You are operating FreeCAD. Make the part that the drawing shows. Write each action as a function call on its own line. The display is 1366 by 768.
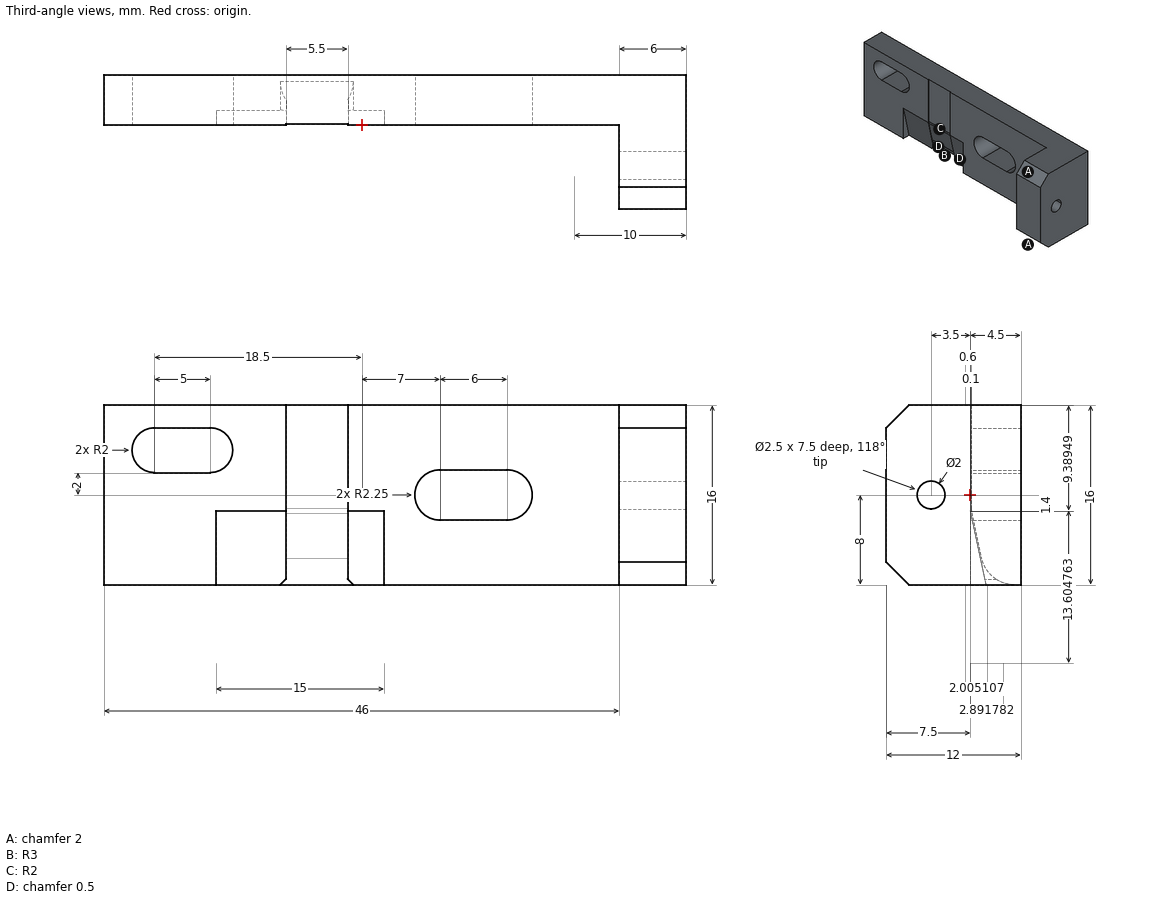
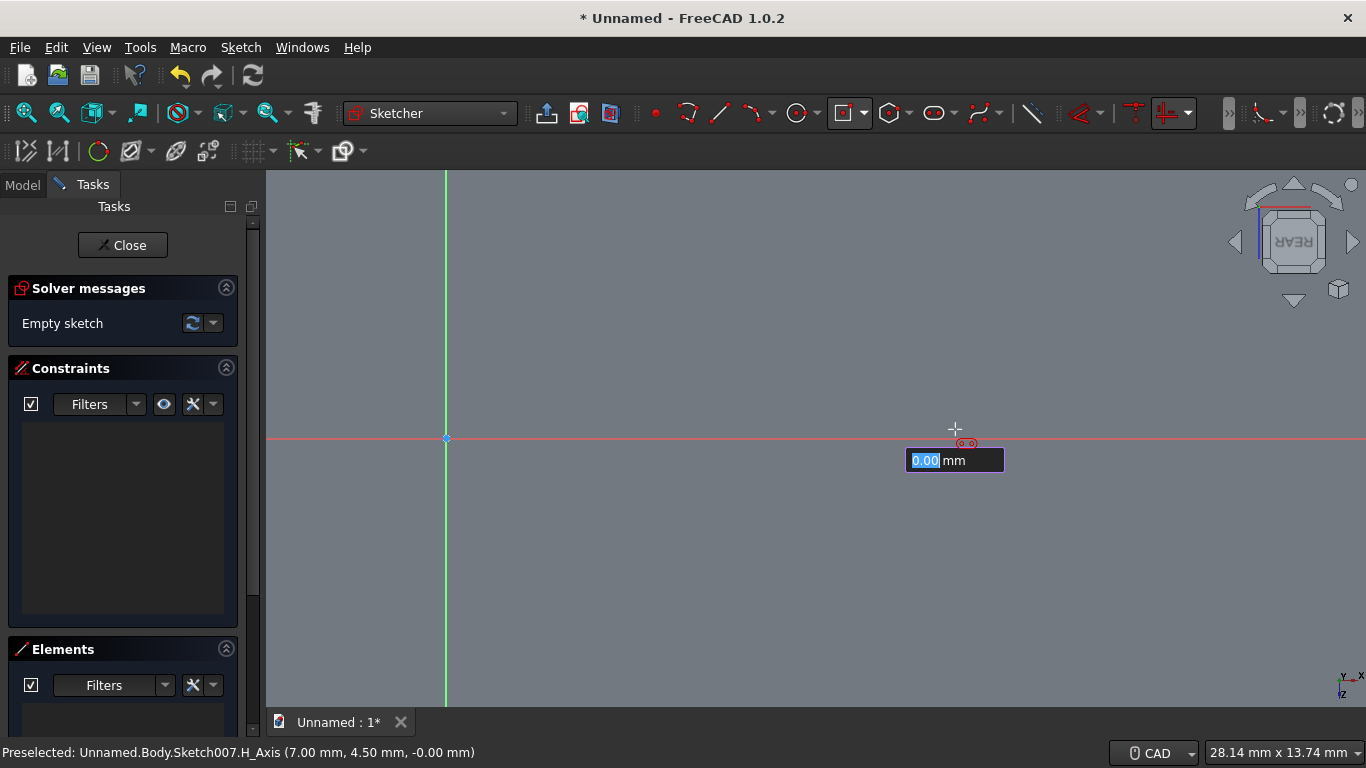
click(837, 351)
key(Escape)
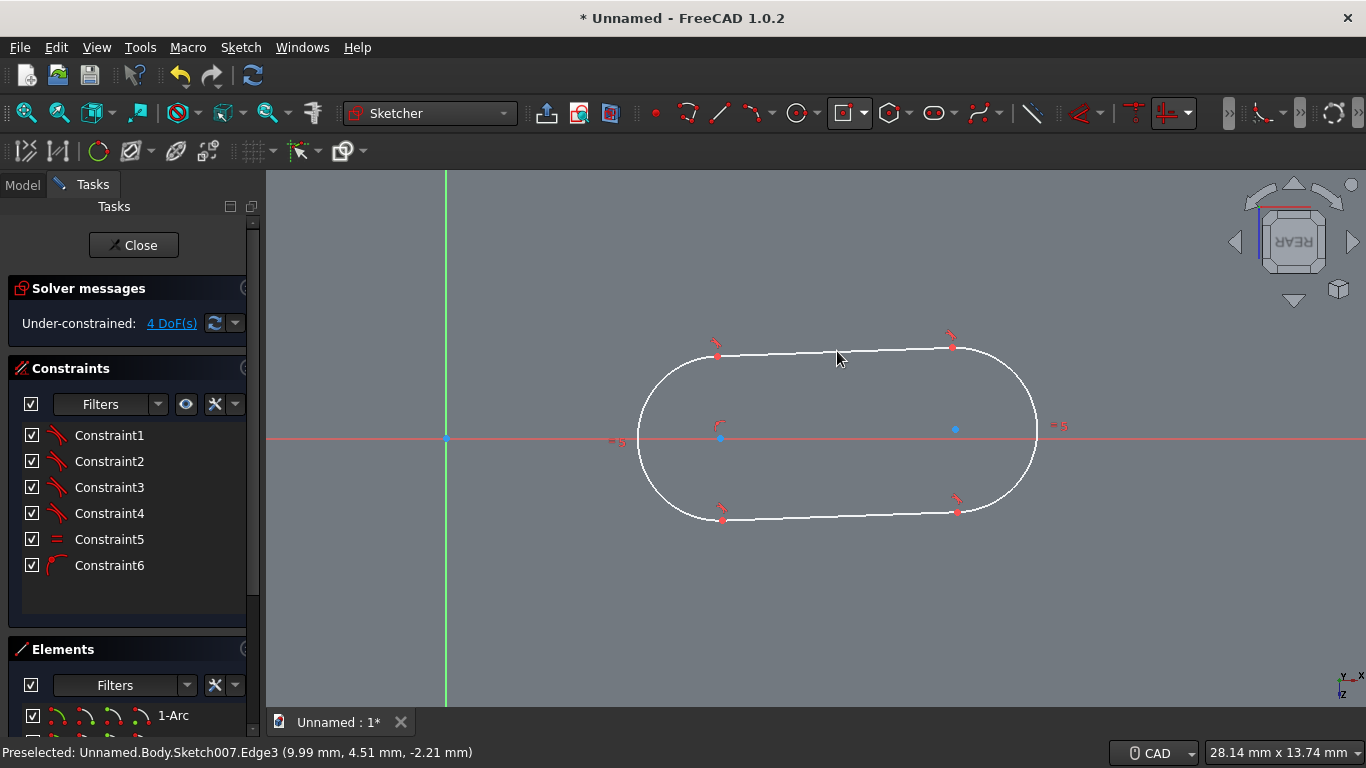
click(788, 354)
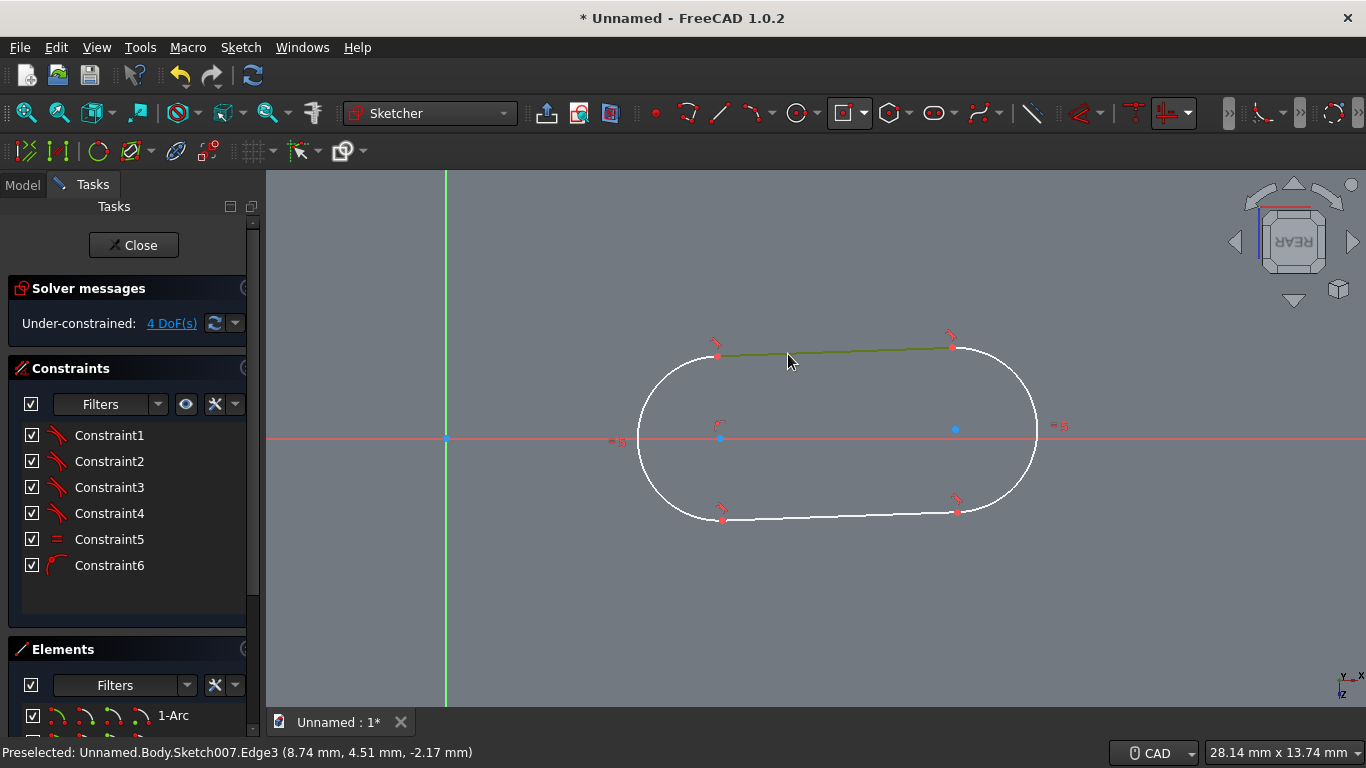
key(h)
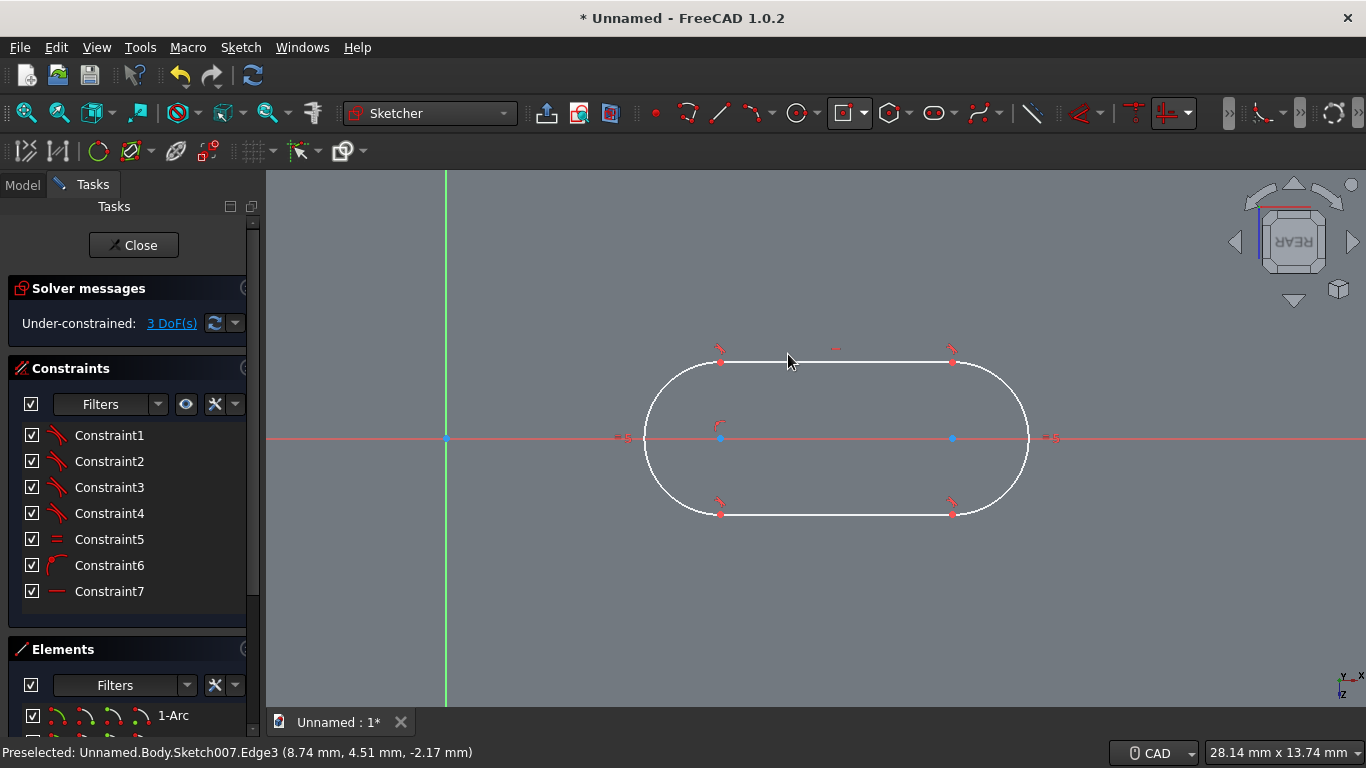
key(d)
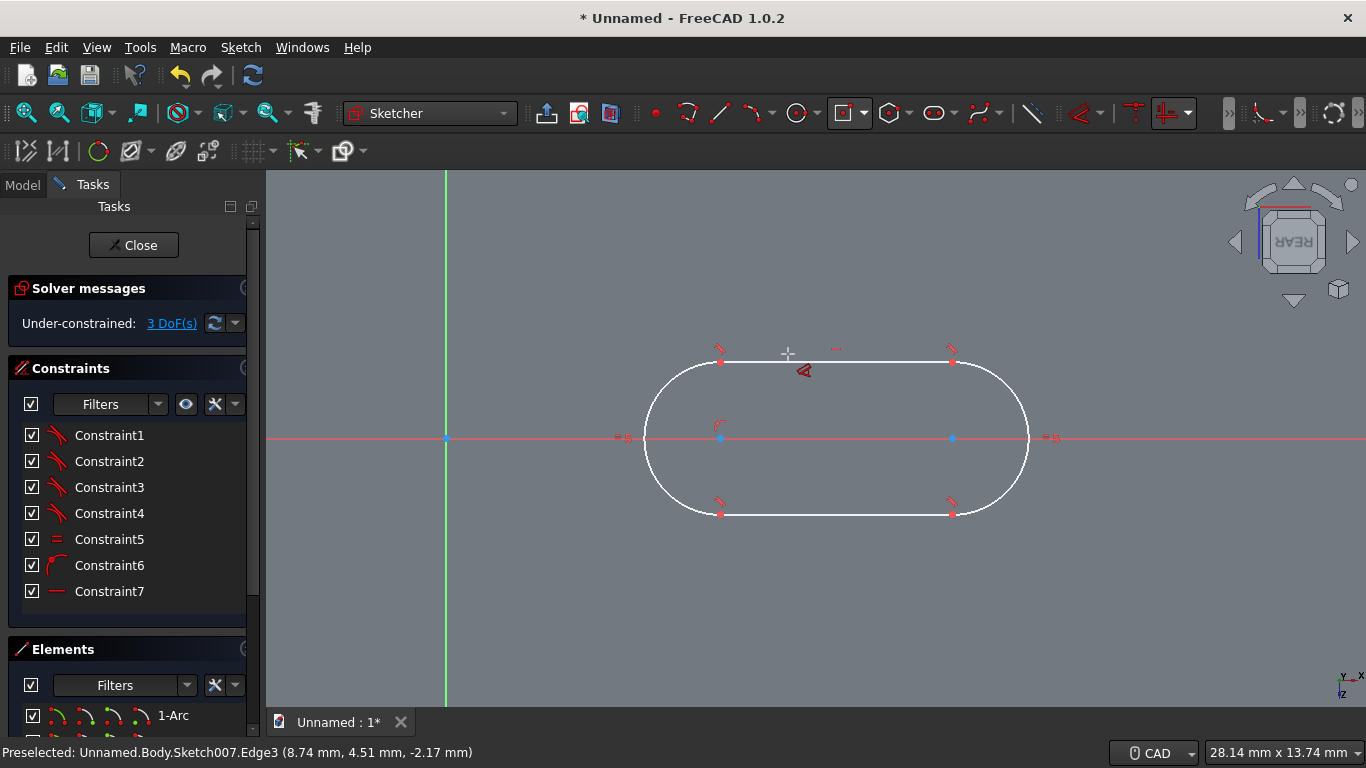
click(659, 394)
click(633, 375)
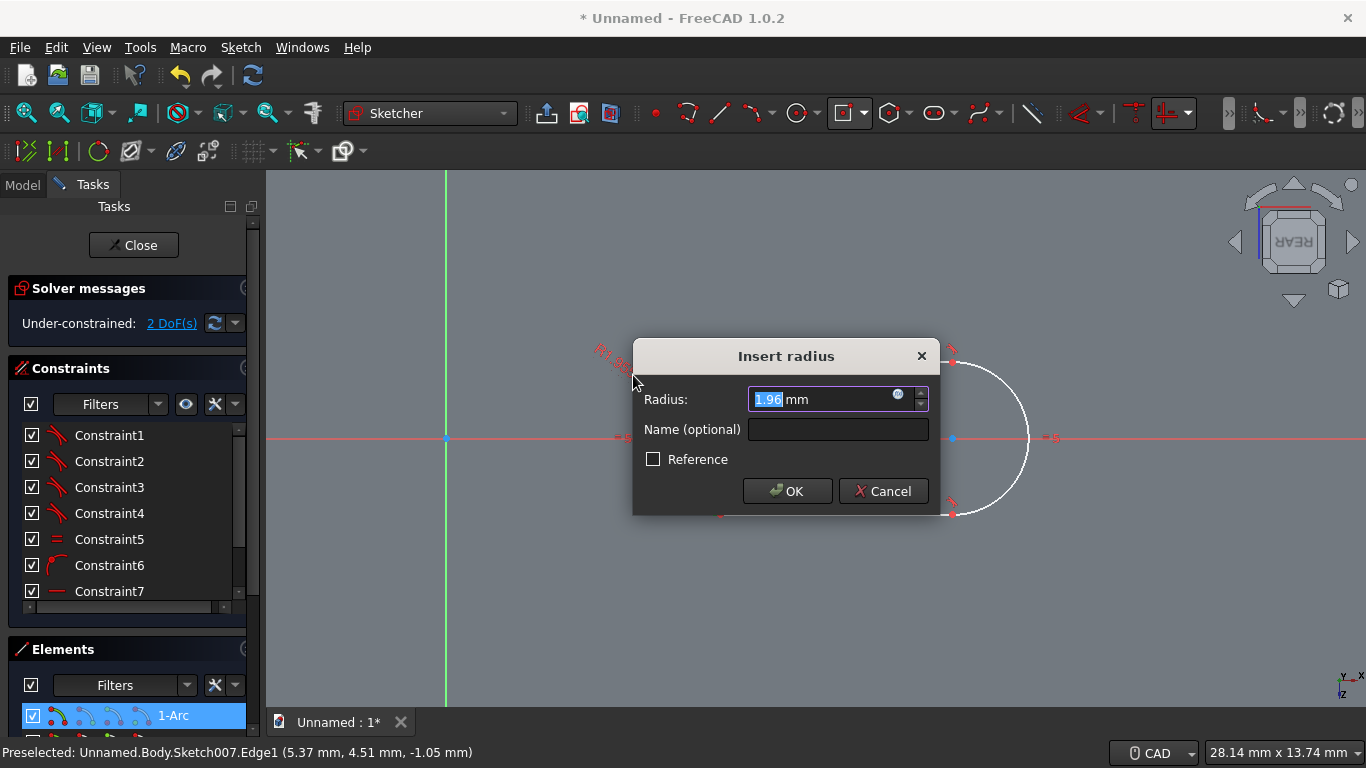
text(2.25)
key(Return)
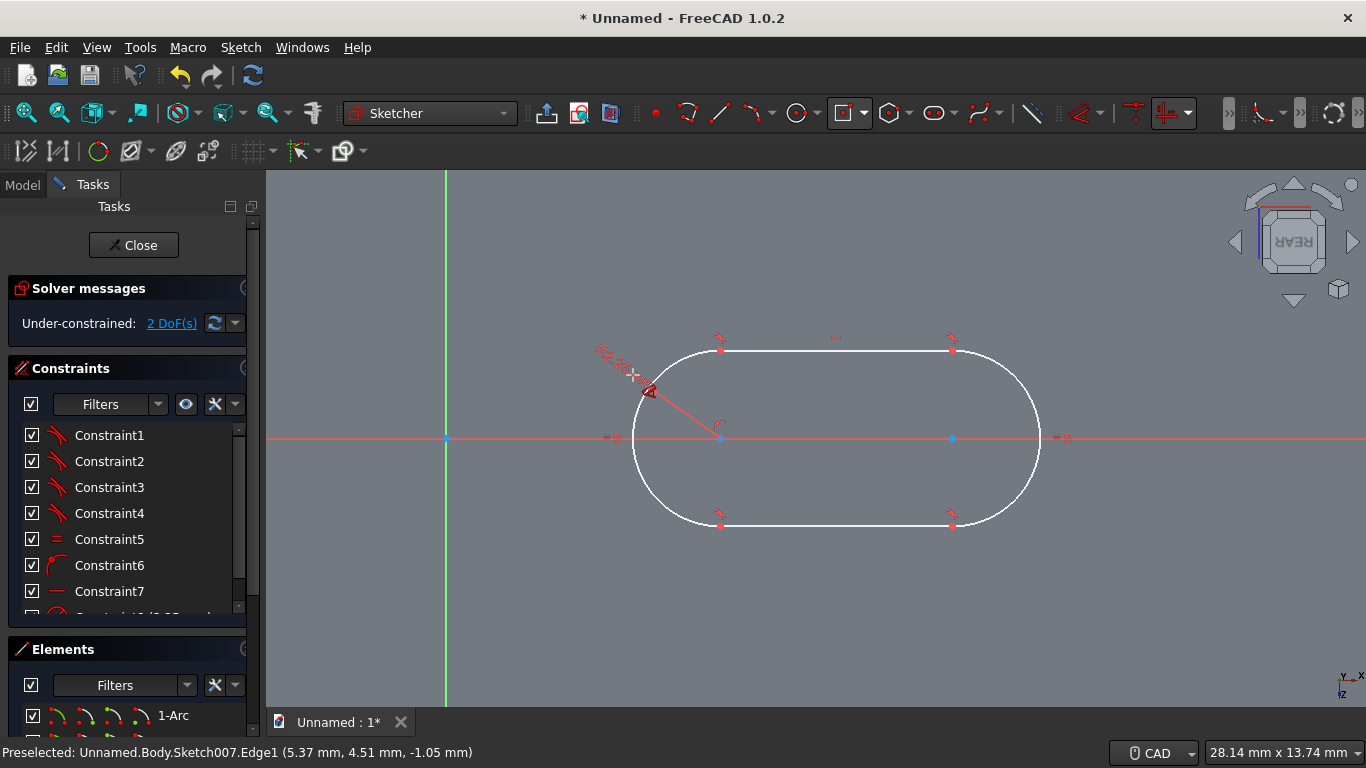
click(790, 351)
click(837, 317)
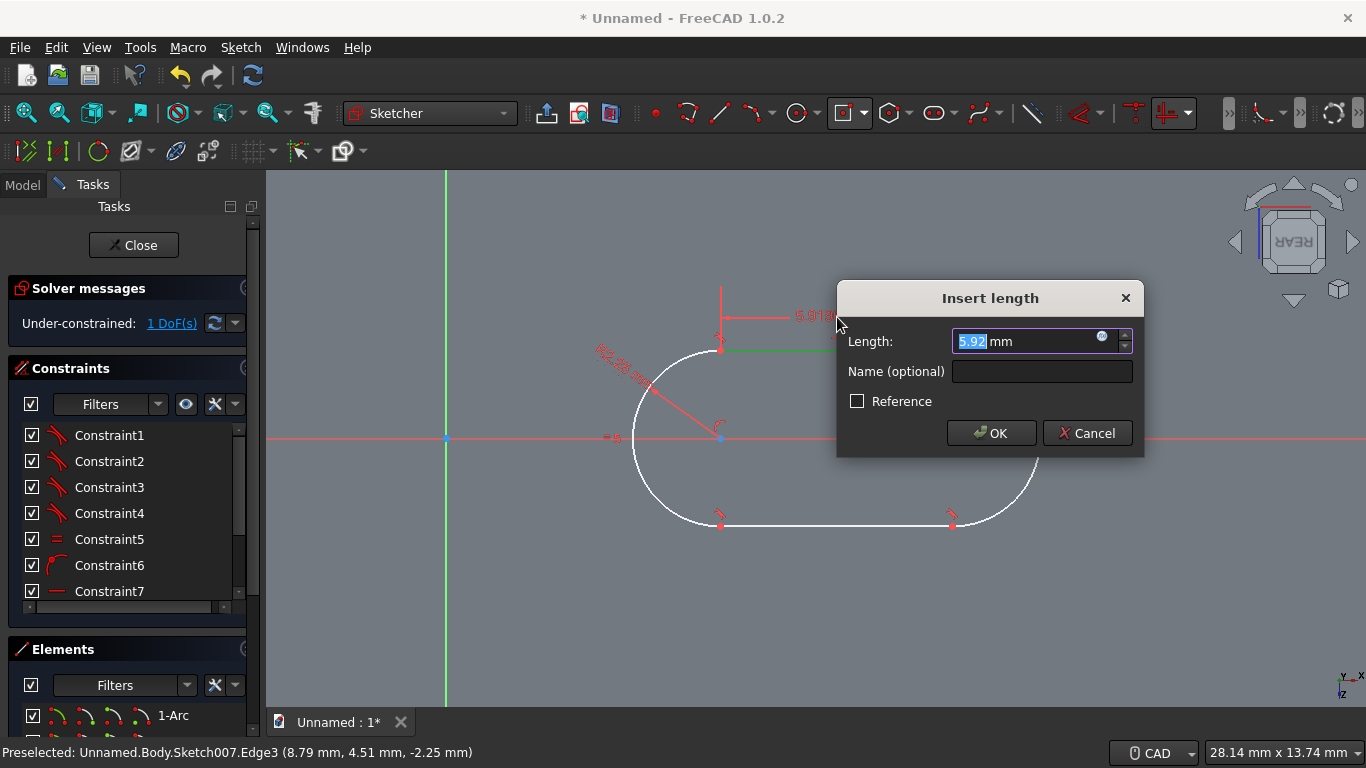
text(6)
key(Return)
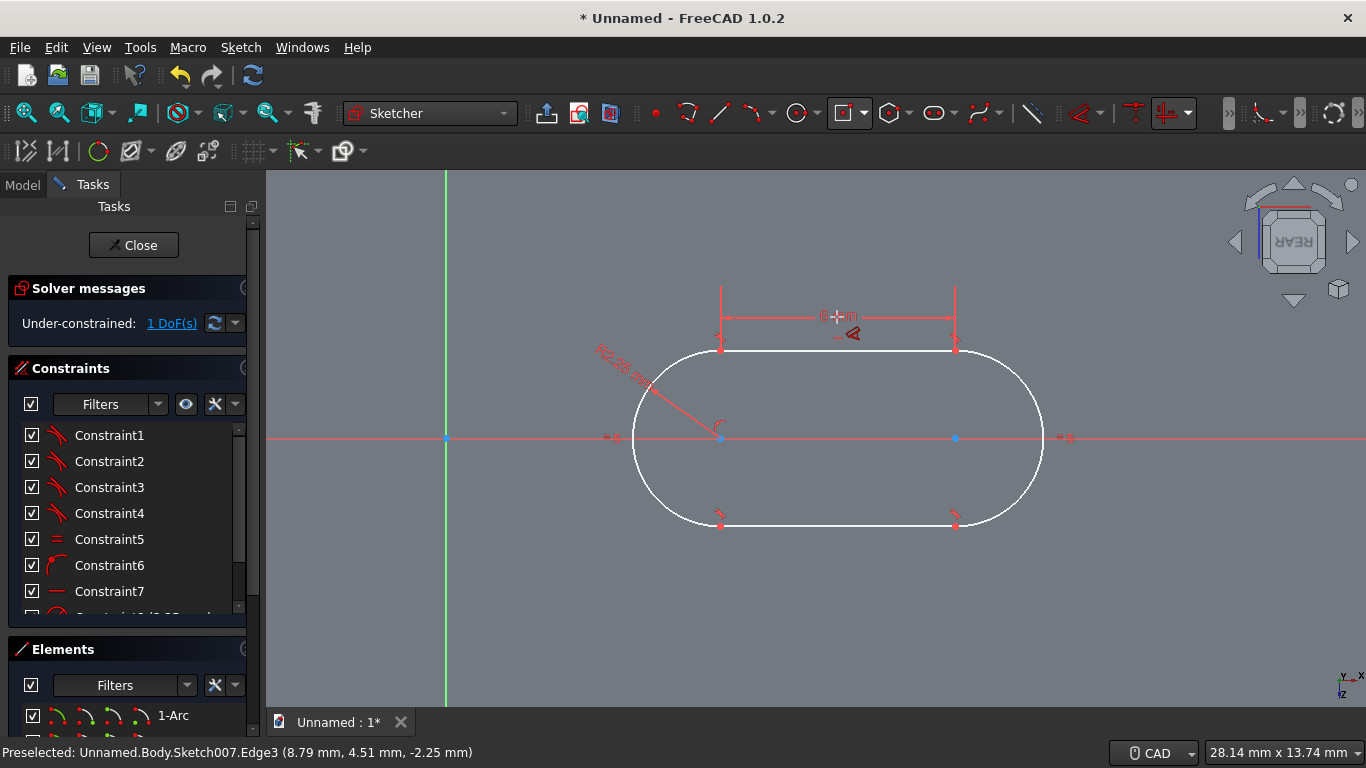
click(721, 351)
click(584, 317)